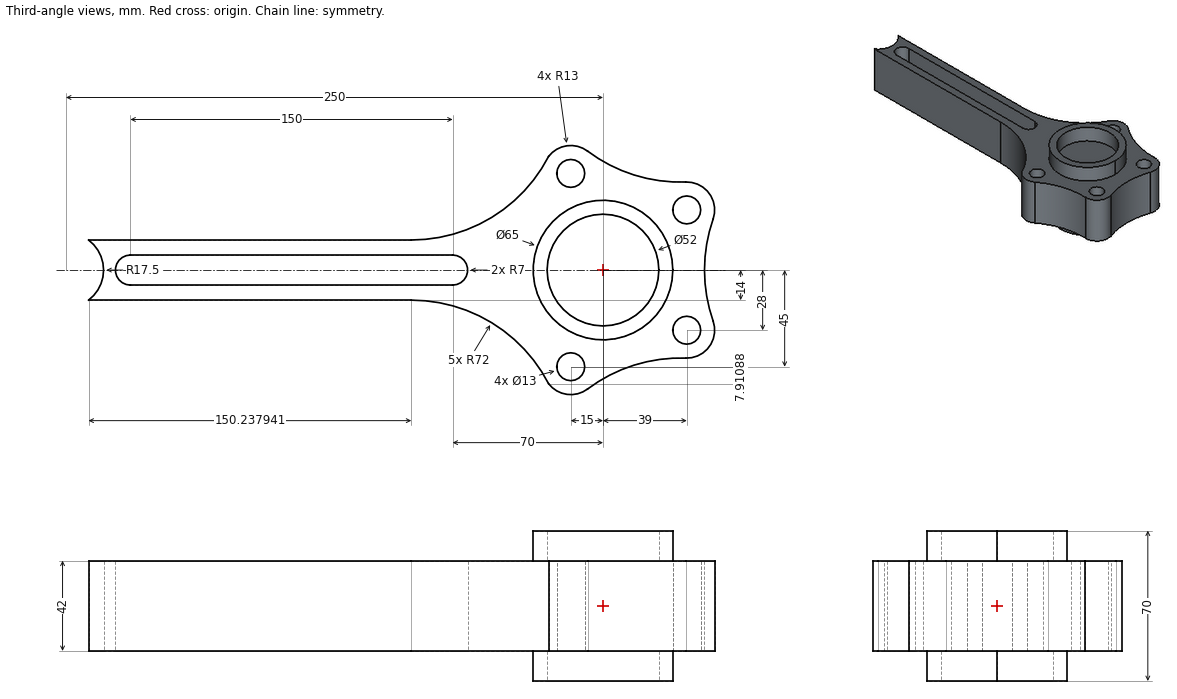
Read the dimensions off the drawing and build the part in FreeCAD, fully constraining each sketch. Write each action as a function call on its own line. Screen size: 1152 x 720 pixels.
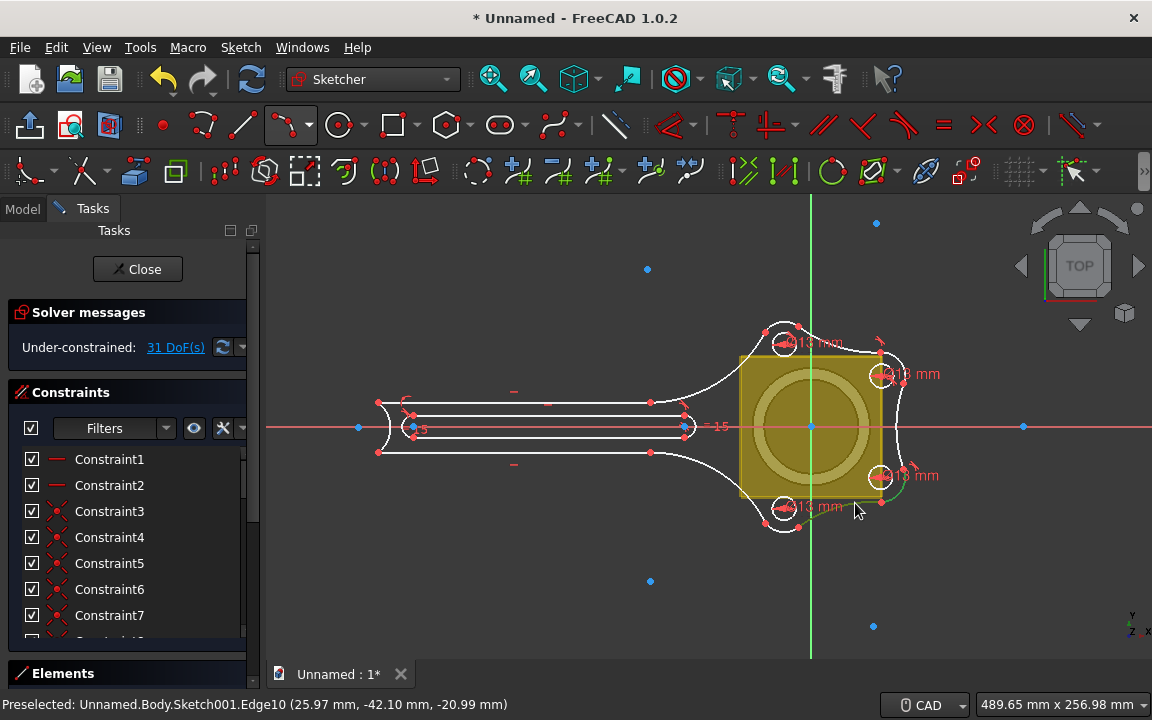
click(904, 126)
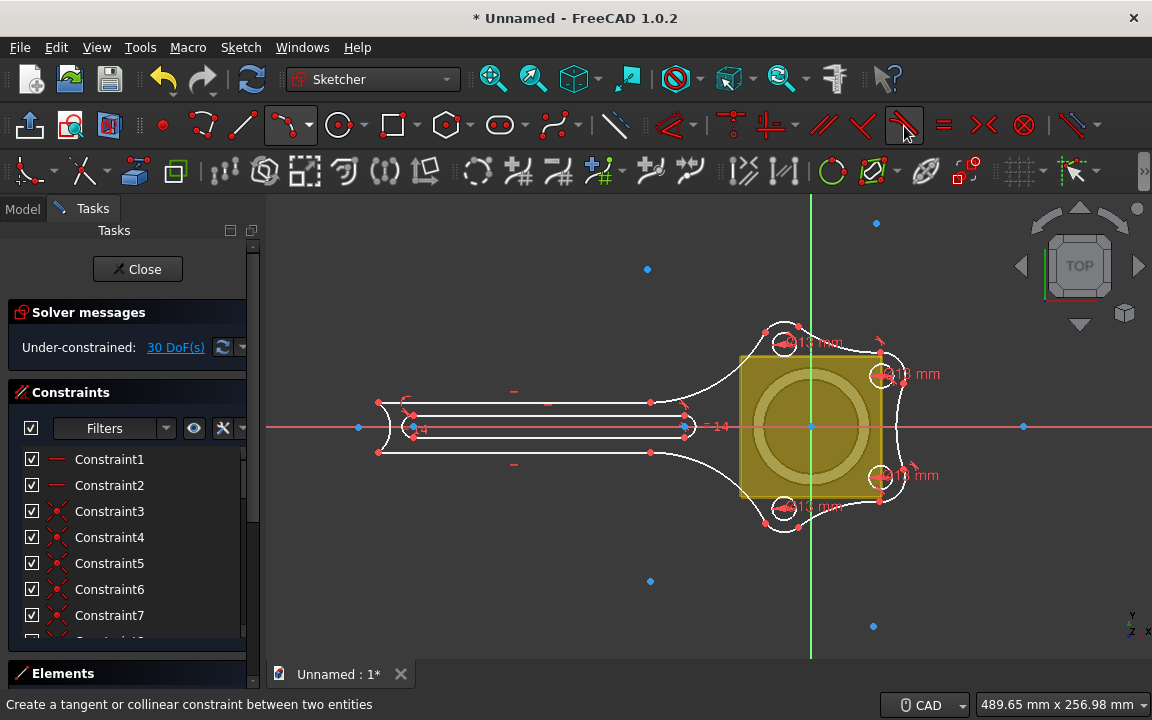
click(854, 504)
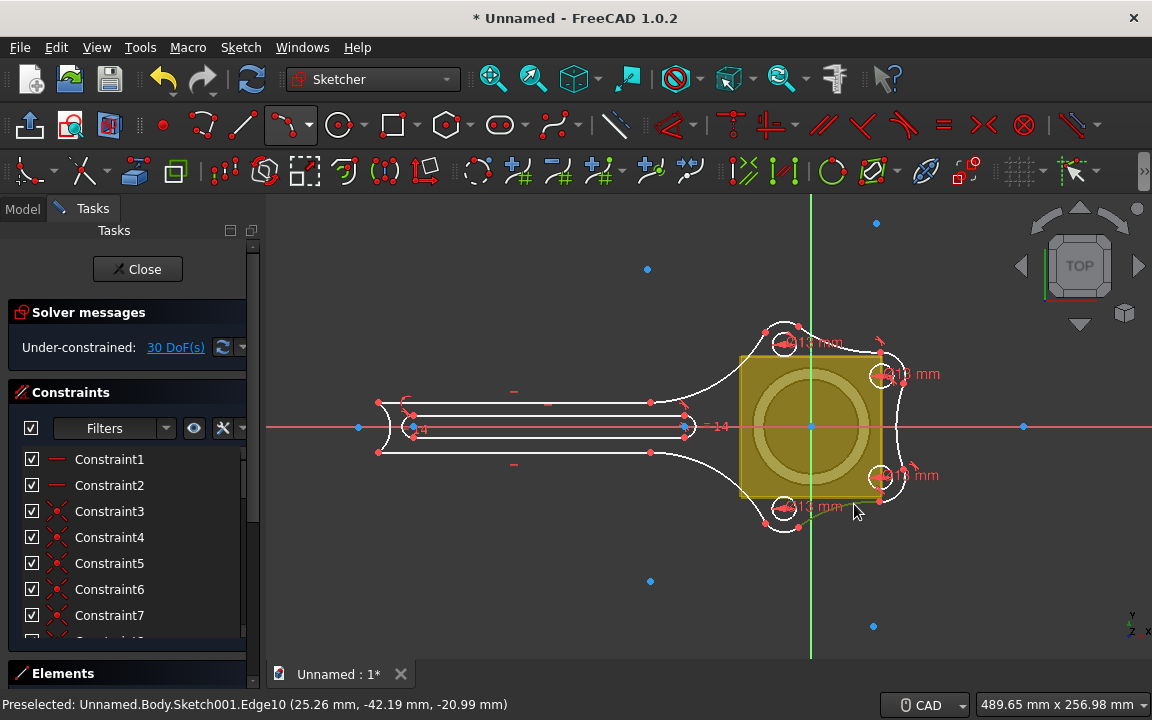
scroll(774, 530, up, 2)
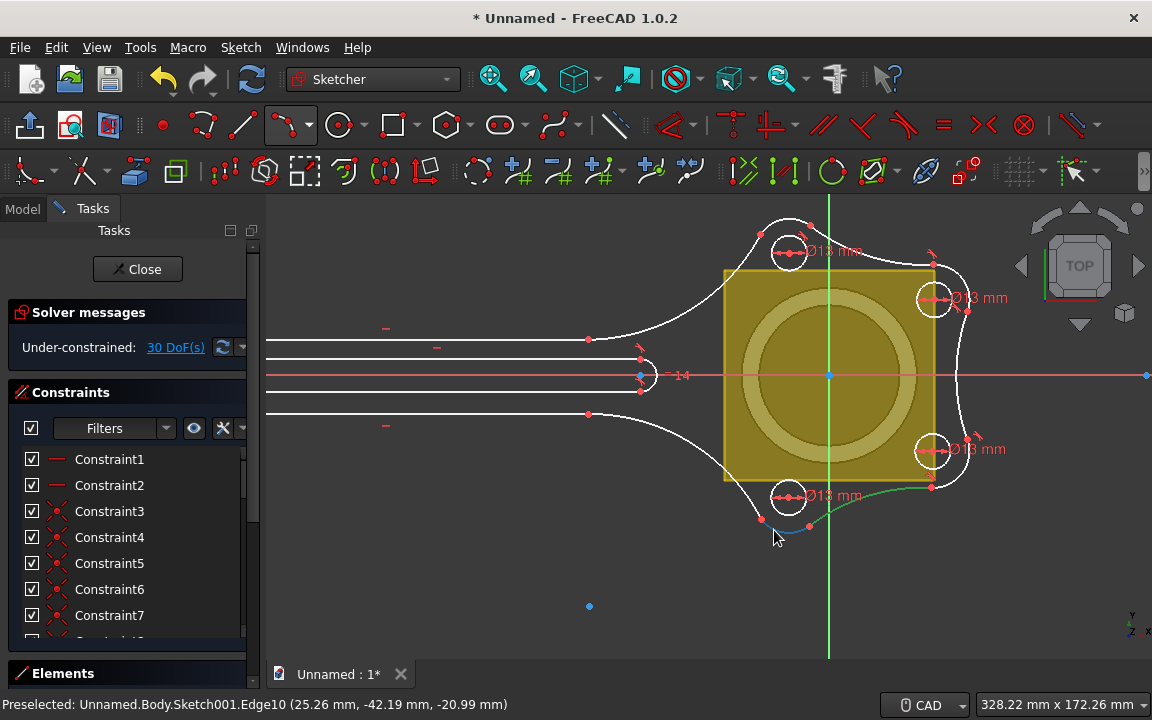
click(774, 529)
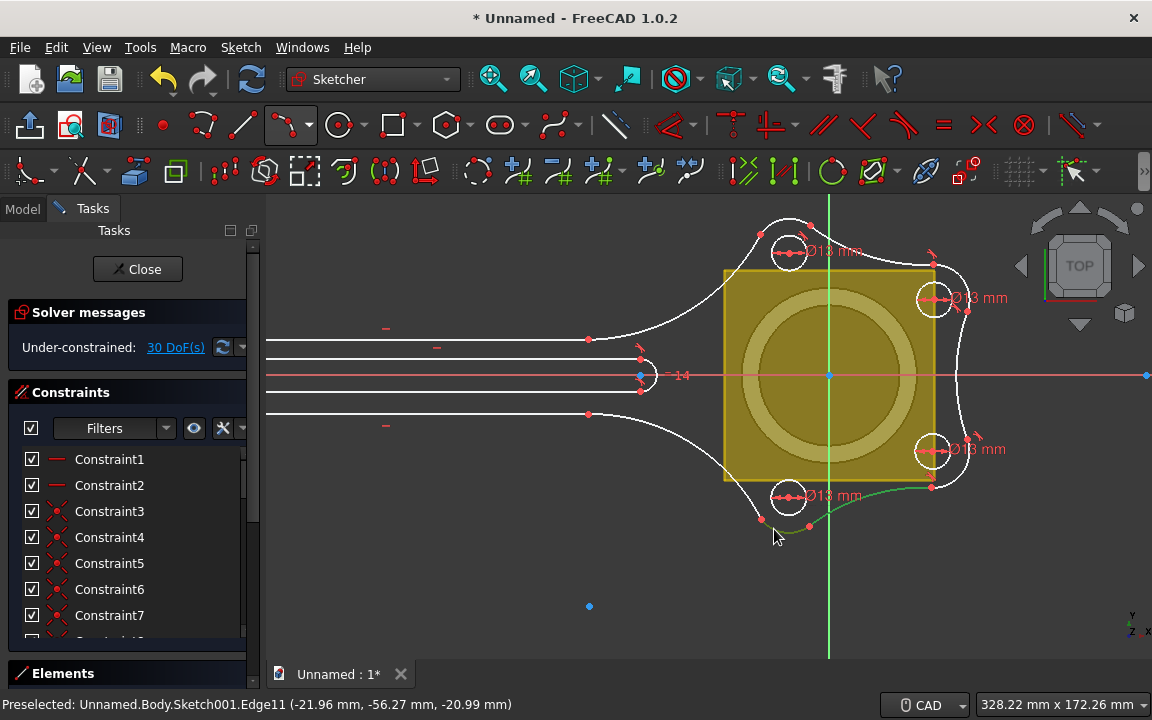
click(904, 126)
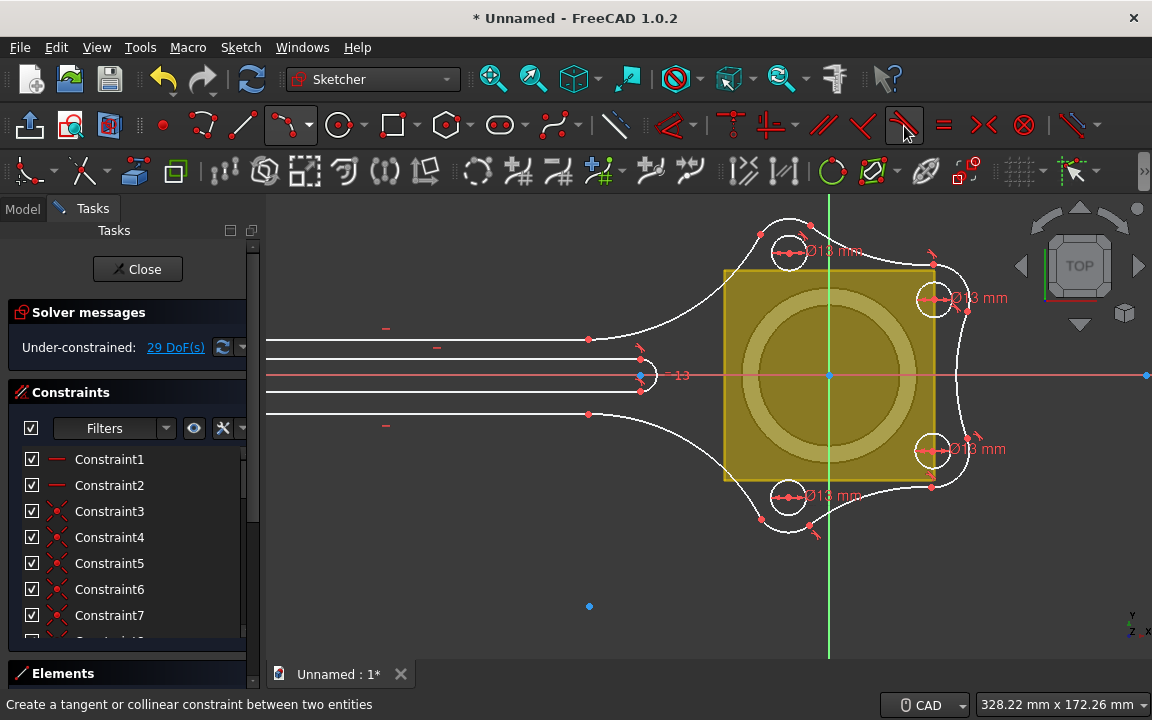
click(651, 329)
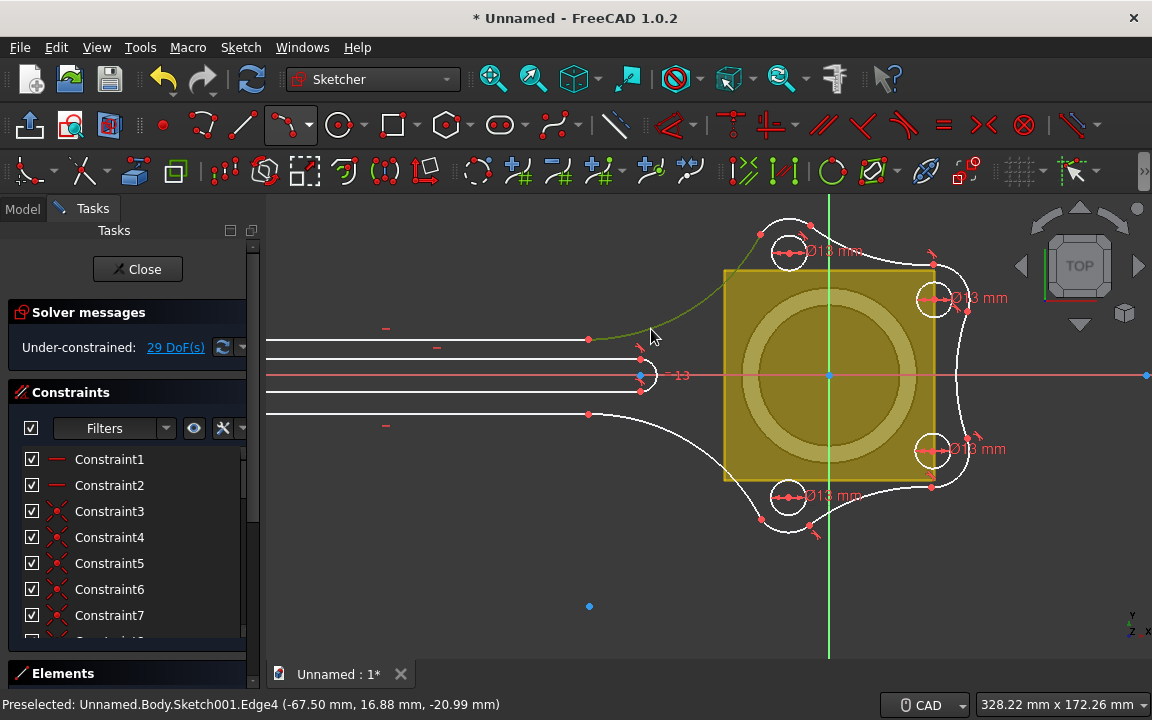
click(844, 246)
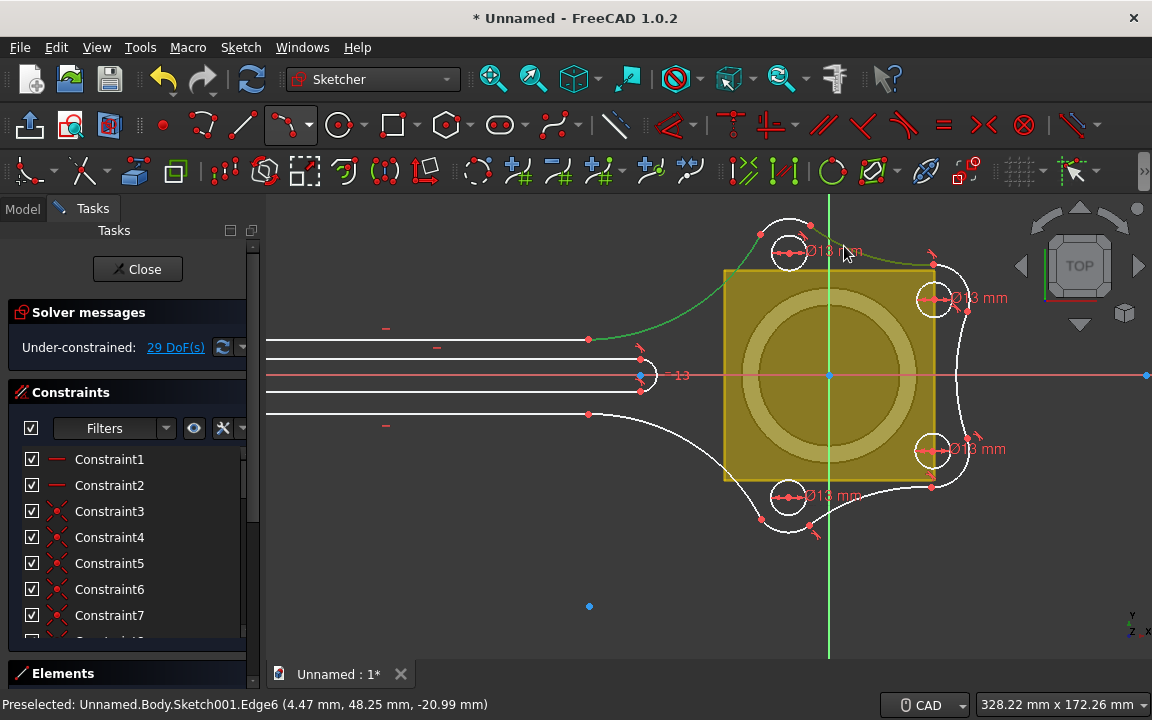
click(958, 349)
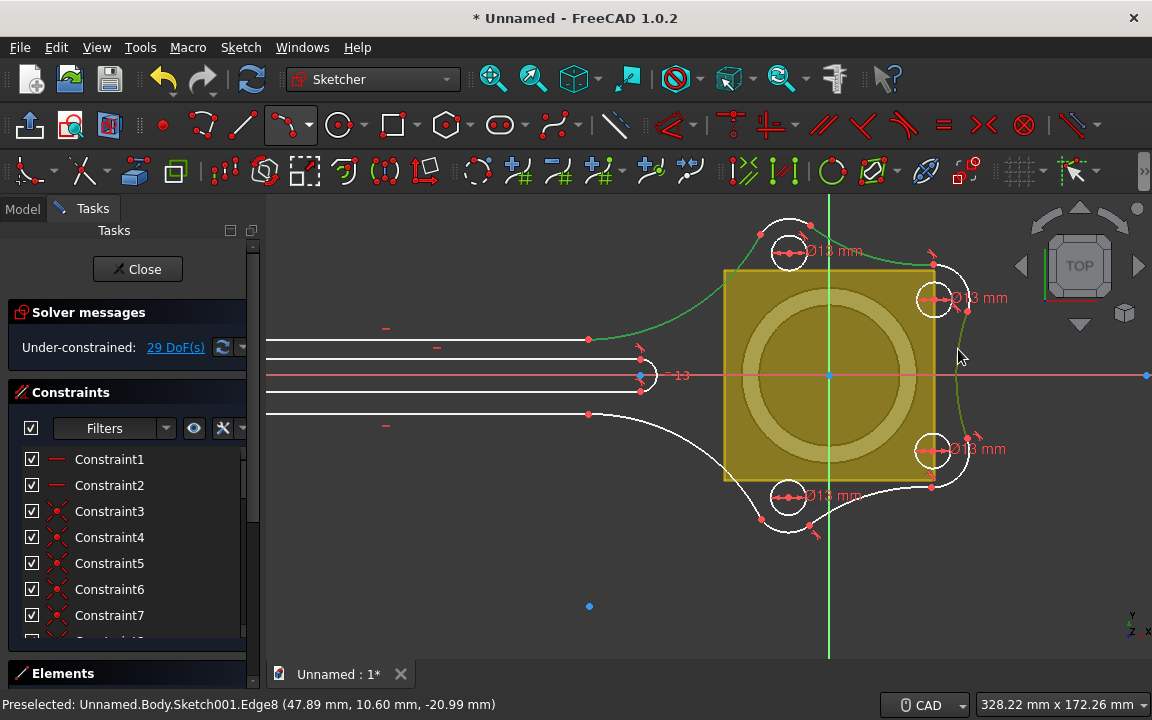
click(892, 490)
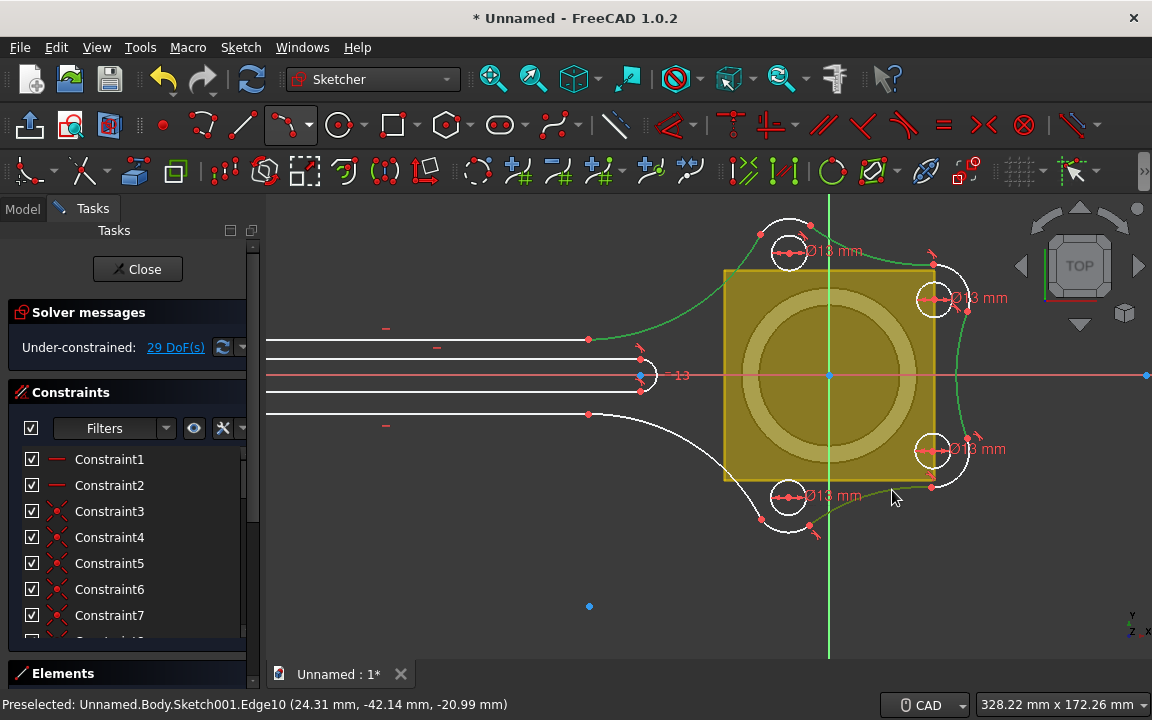
click(724, 468)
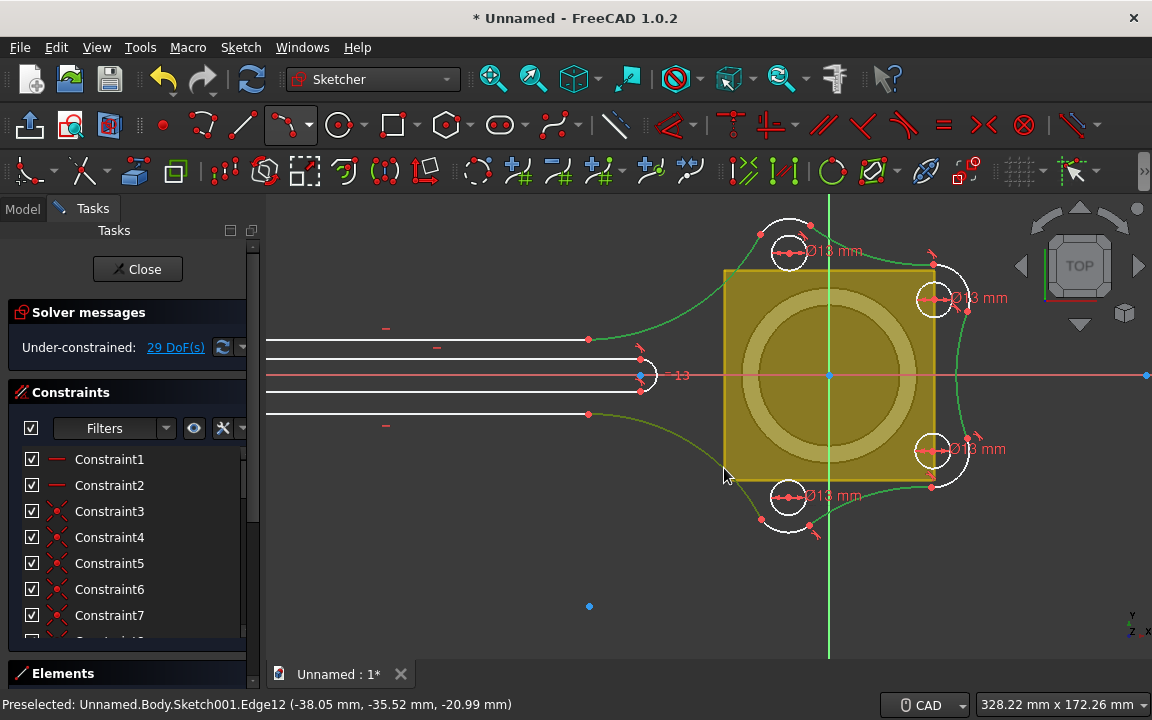
click(944, 126)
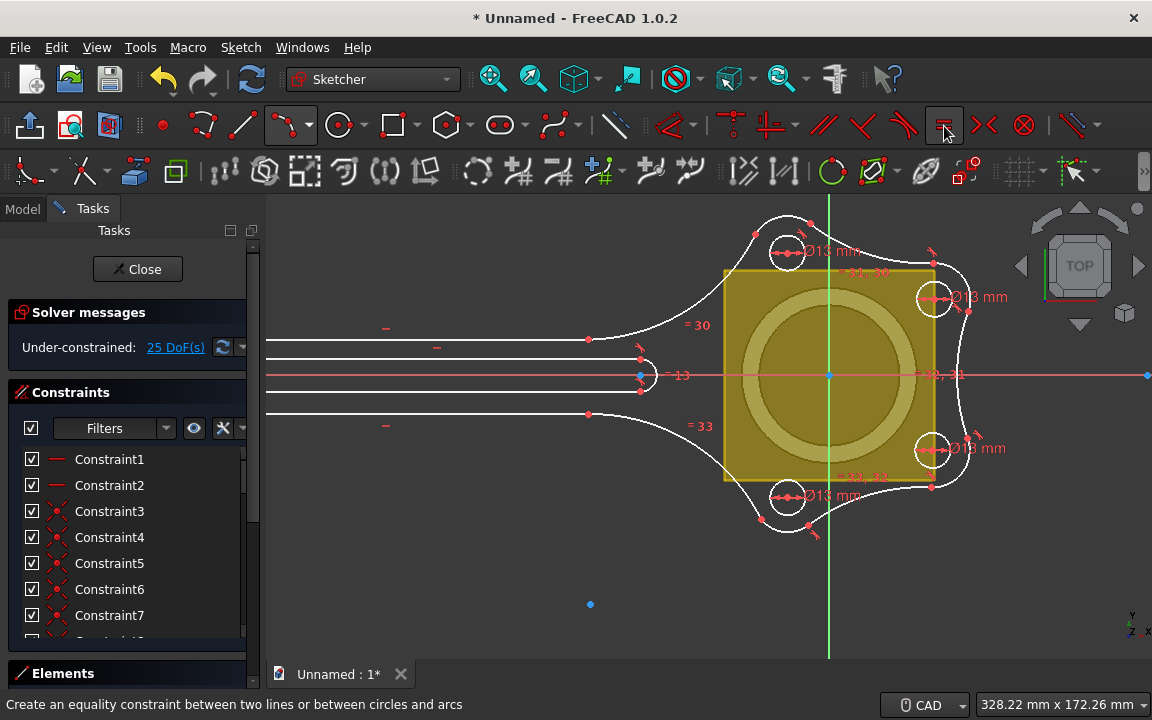
click(764, 225)